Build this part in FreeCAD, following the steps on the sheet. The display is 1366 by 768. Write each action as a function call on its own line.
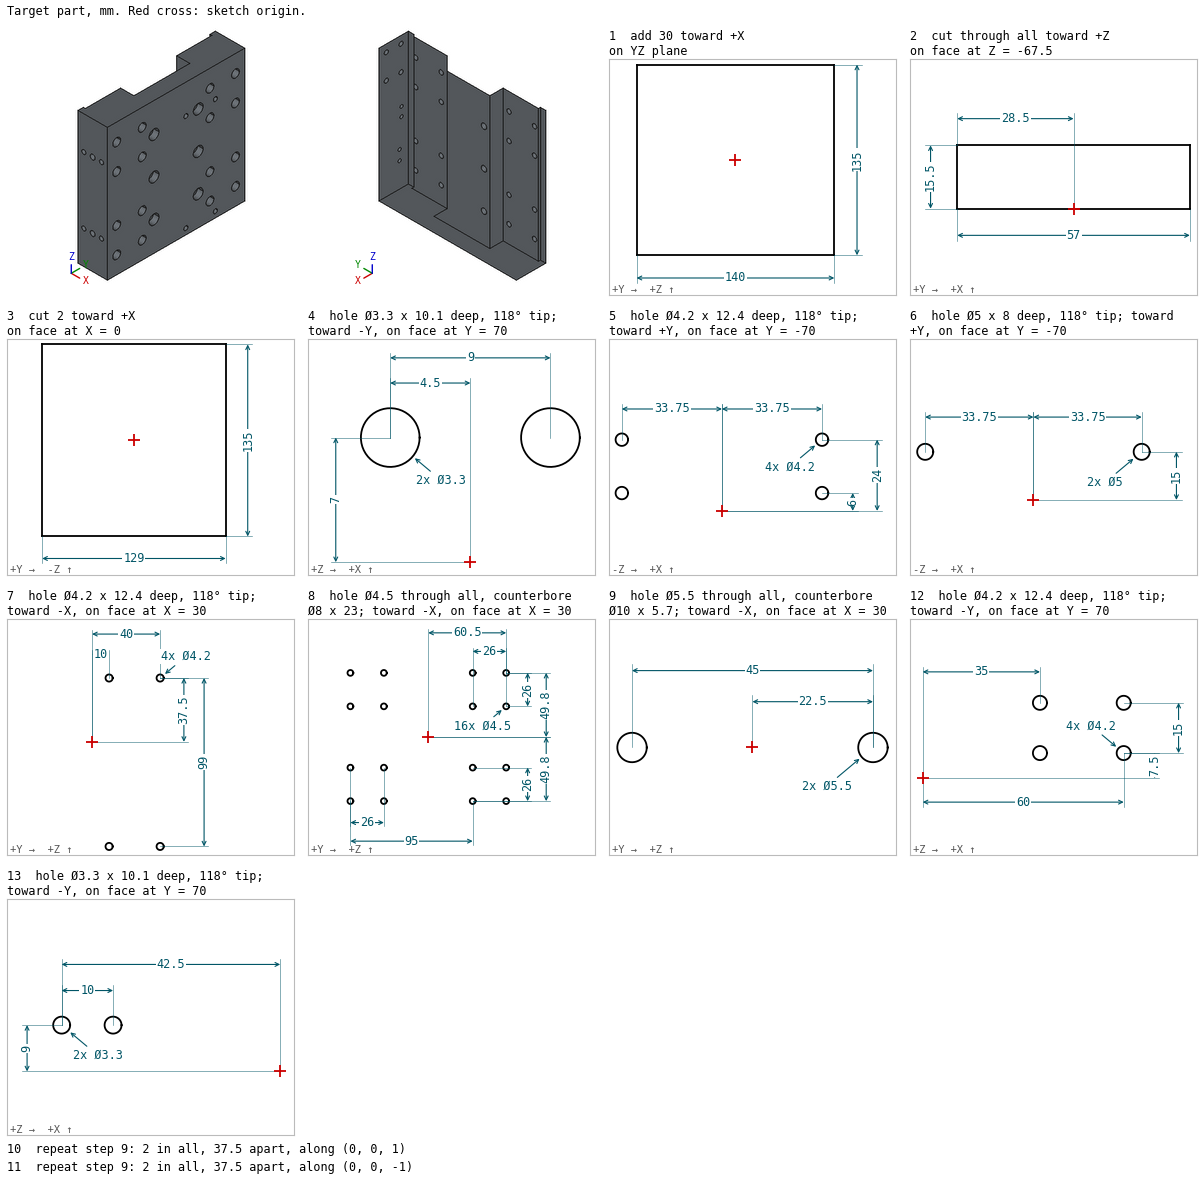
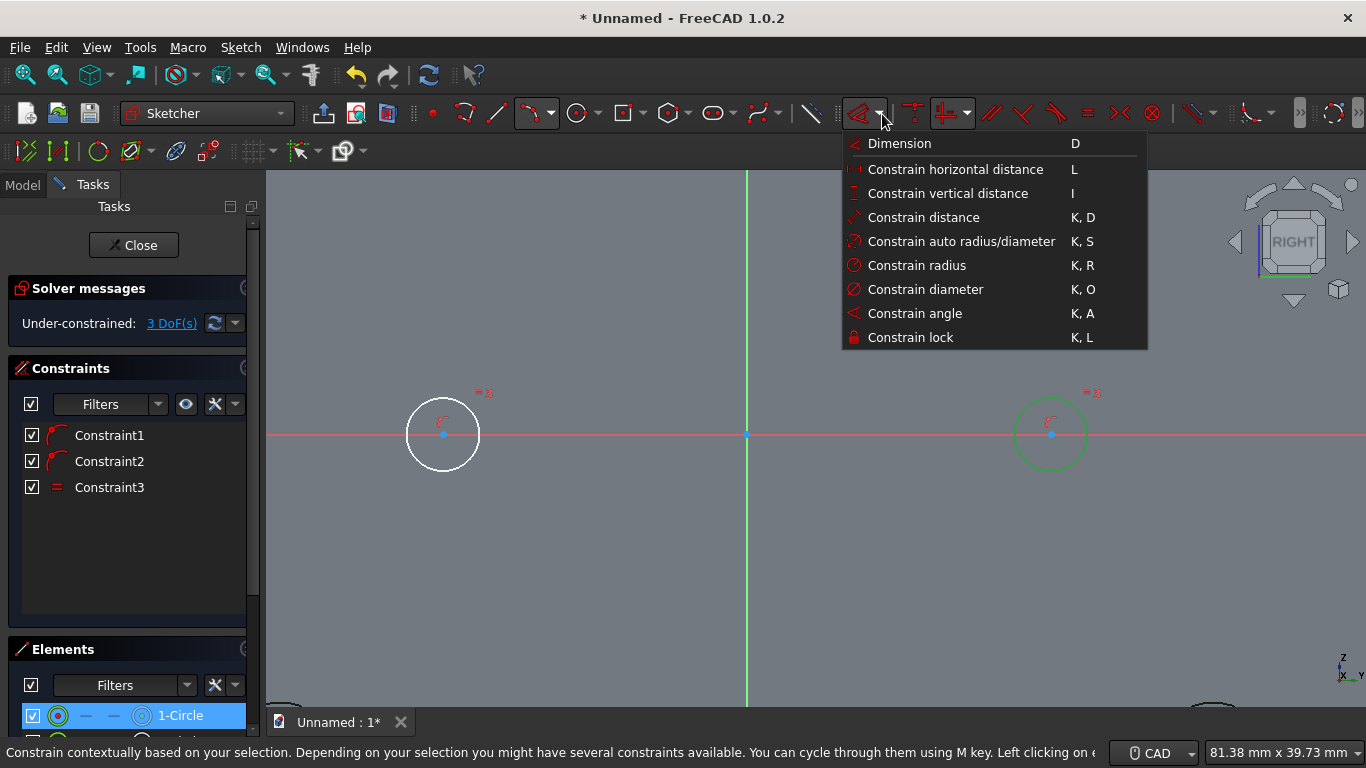
click(995, 289)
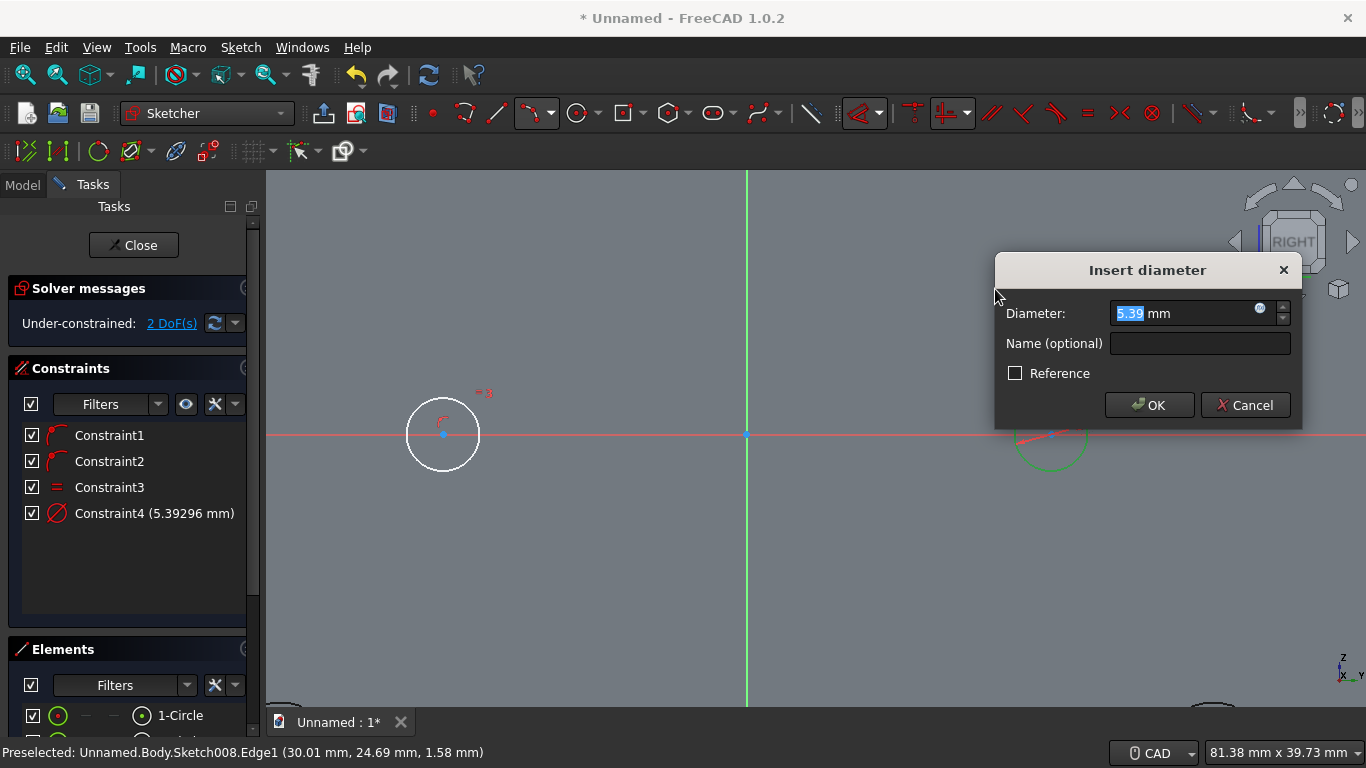
text(5.5)
key(Return)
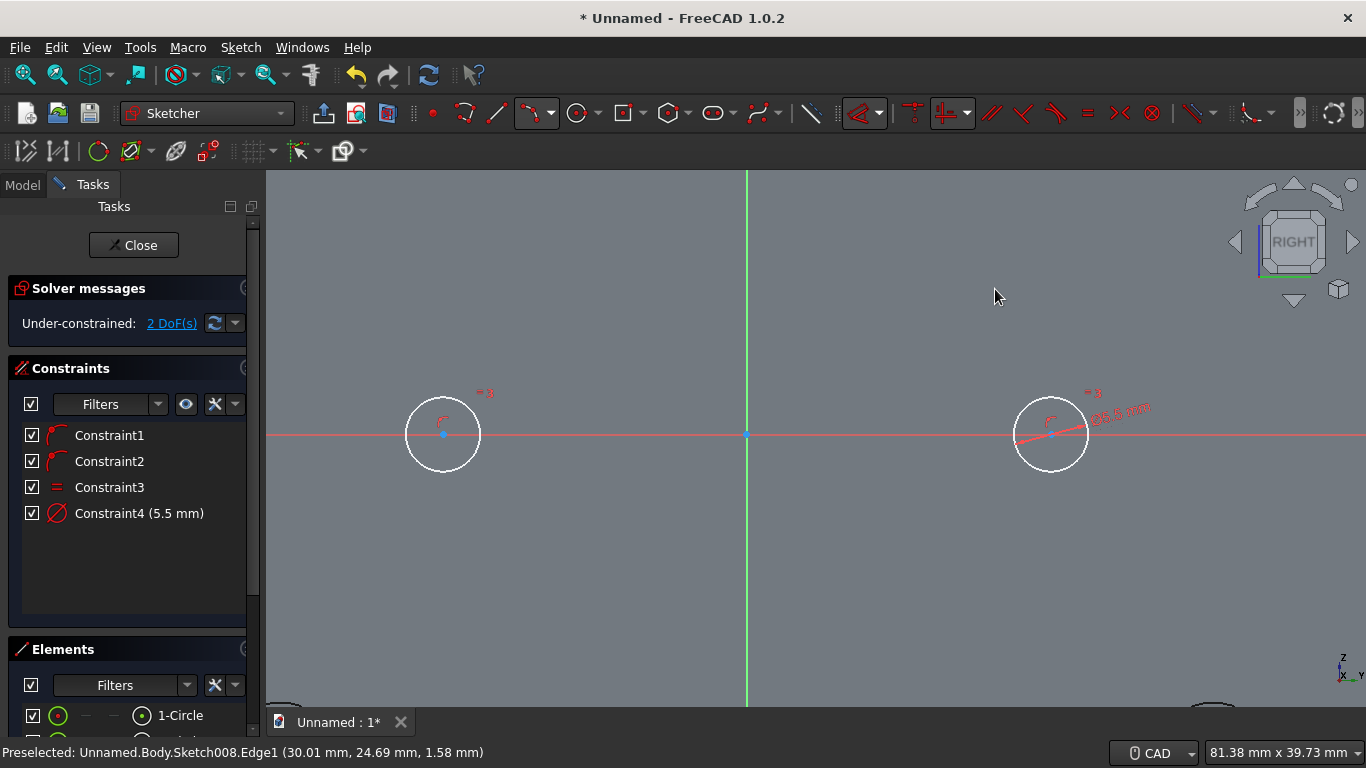
click(1051, 435)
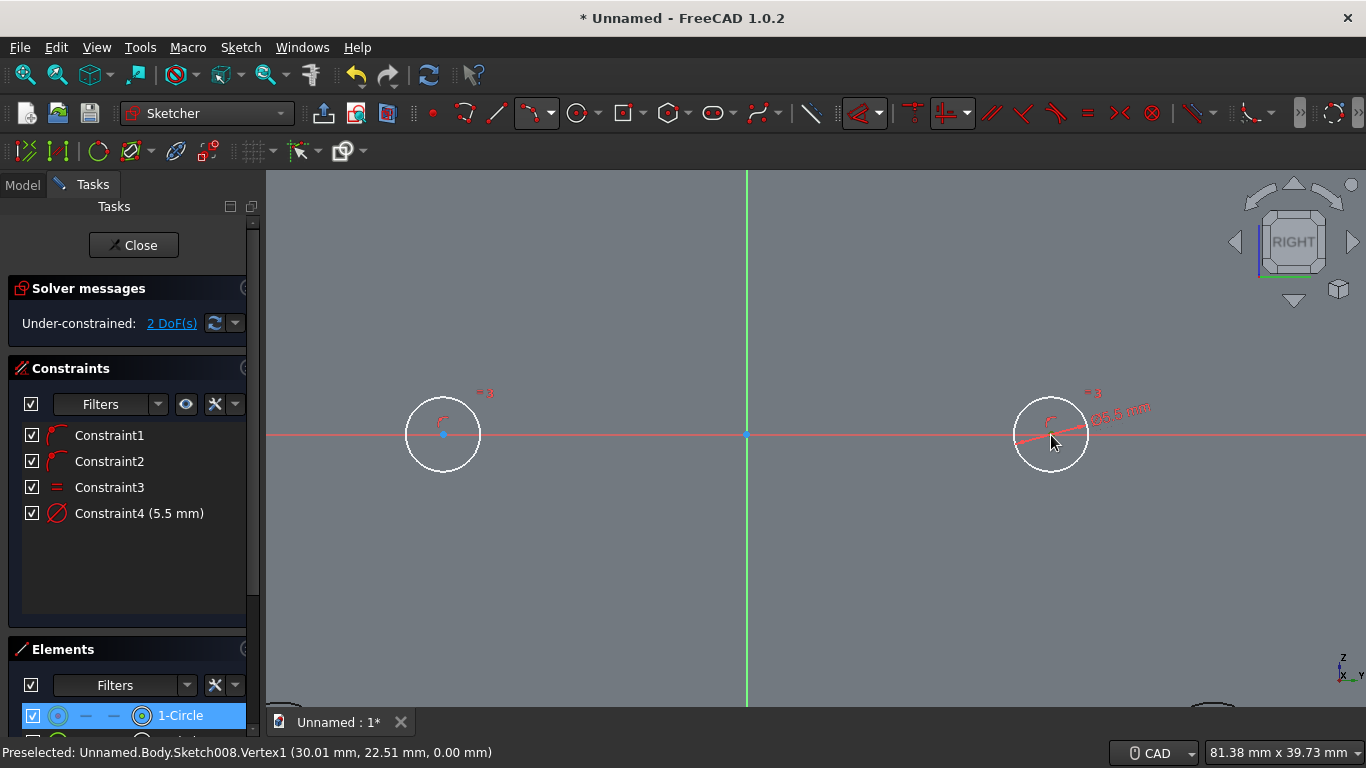
click(443, 435)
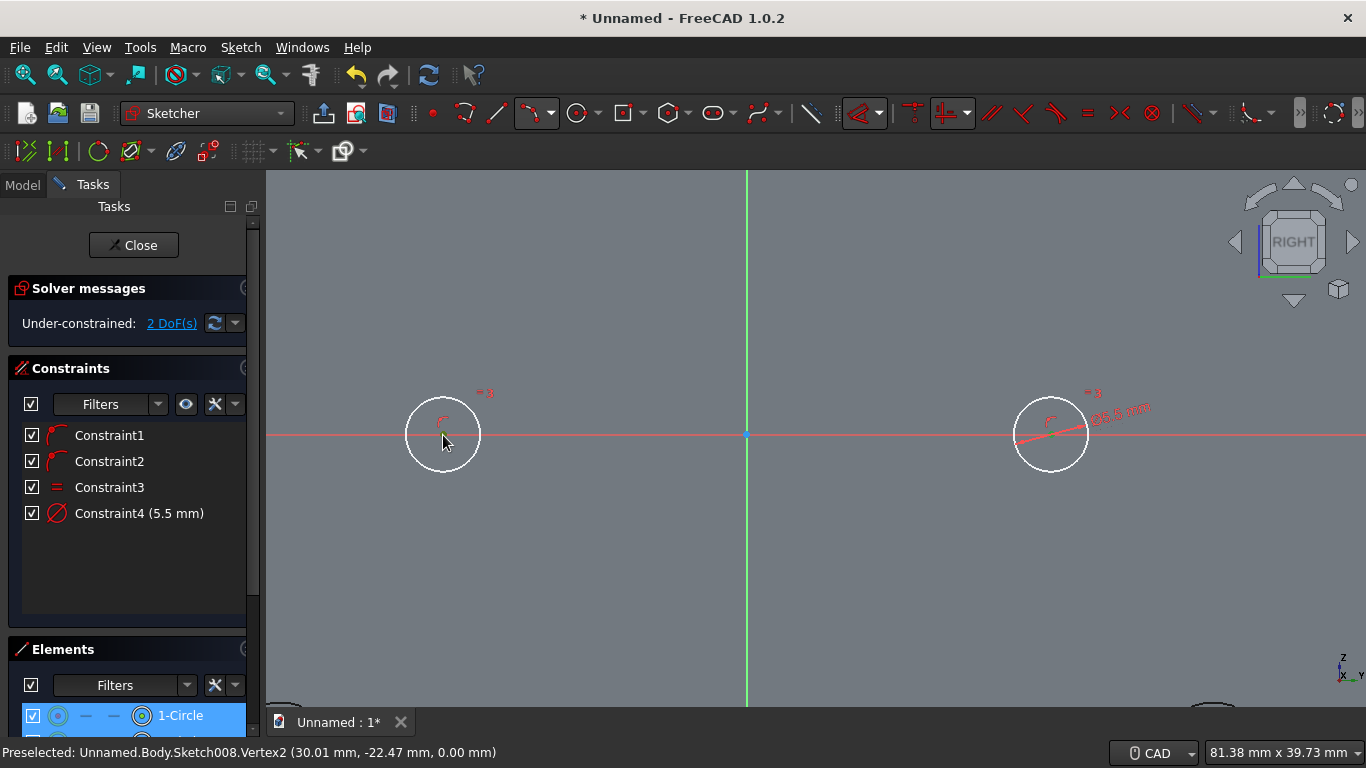
click(882, 114)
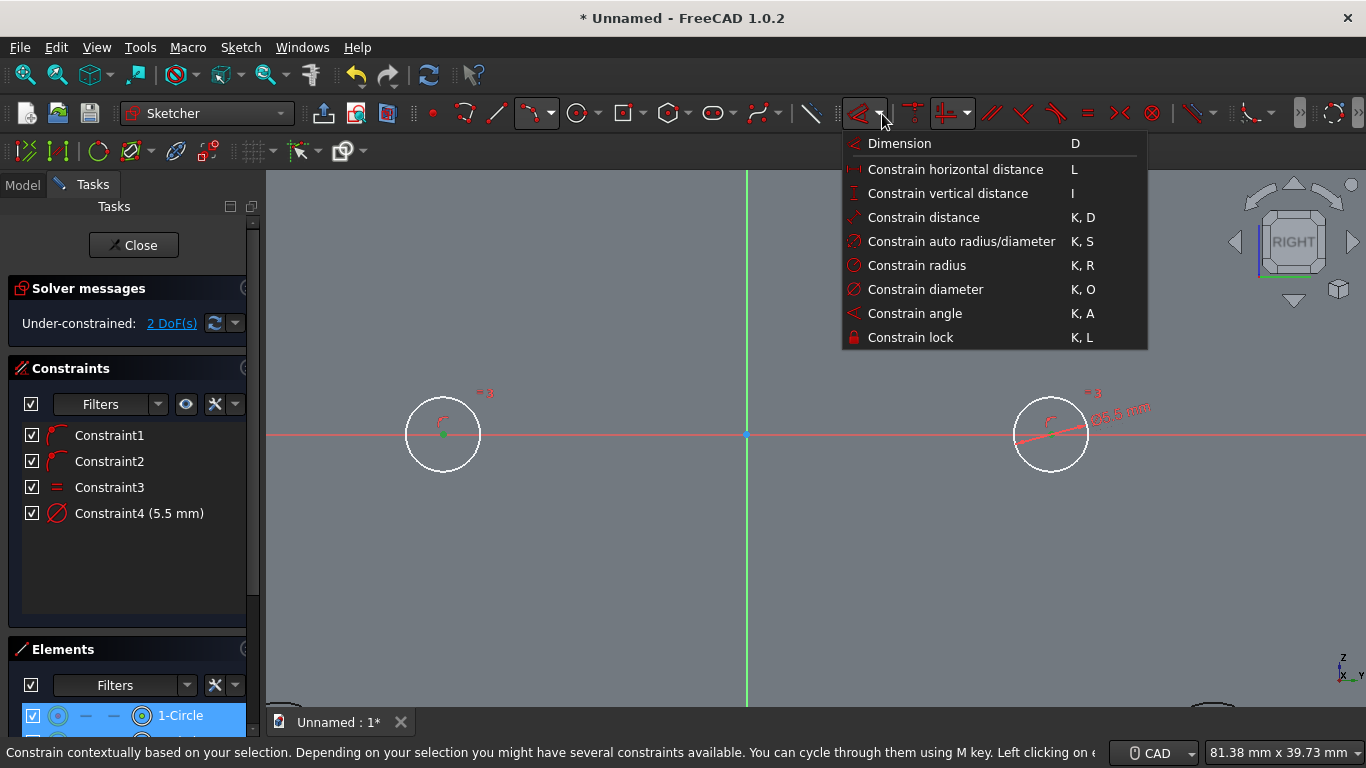
click(995, 169)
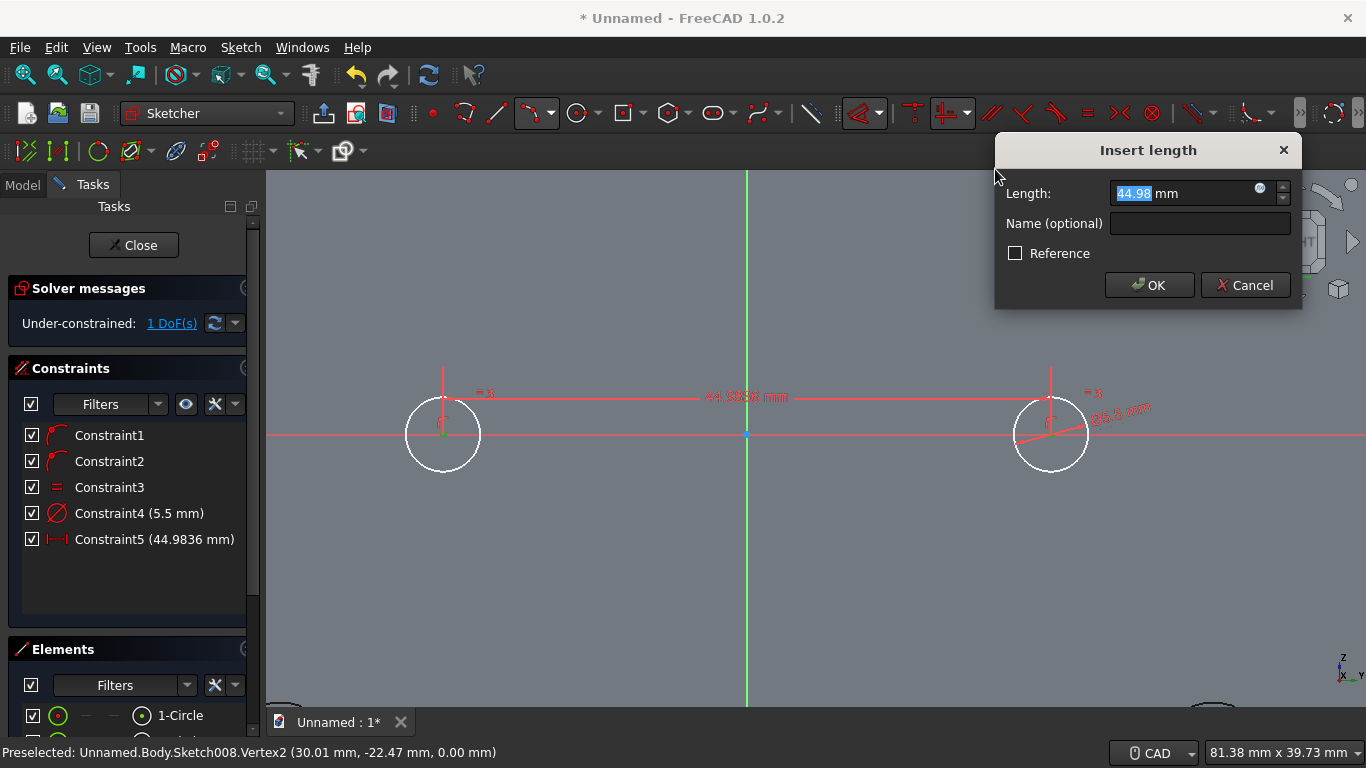
text(45)
key(Return)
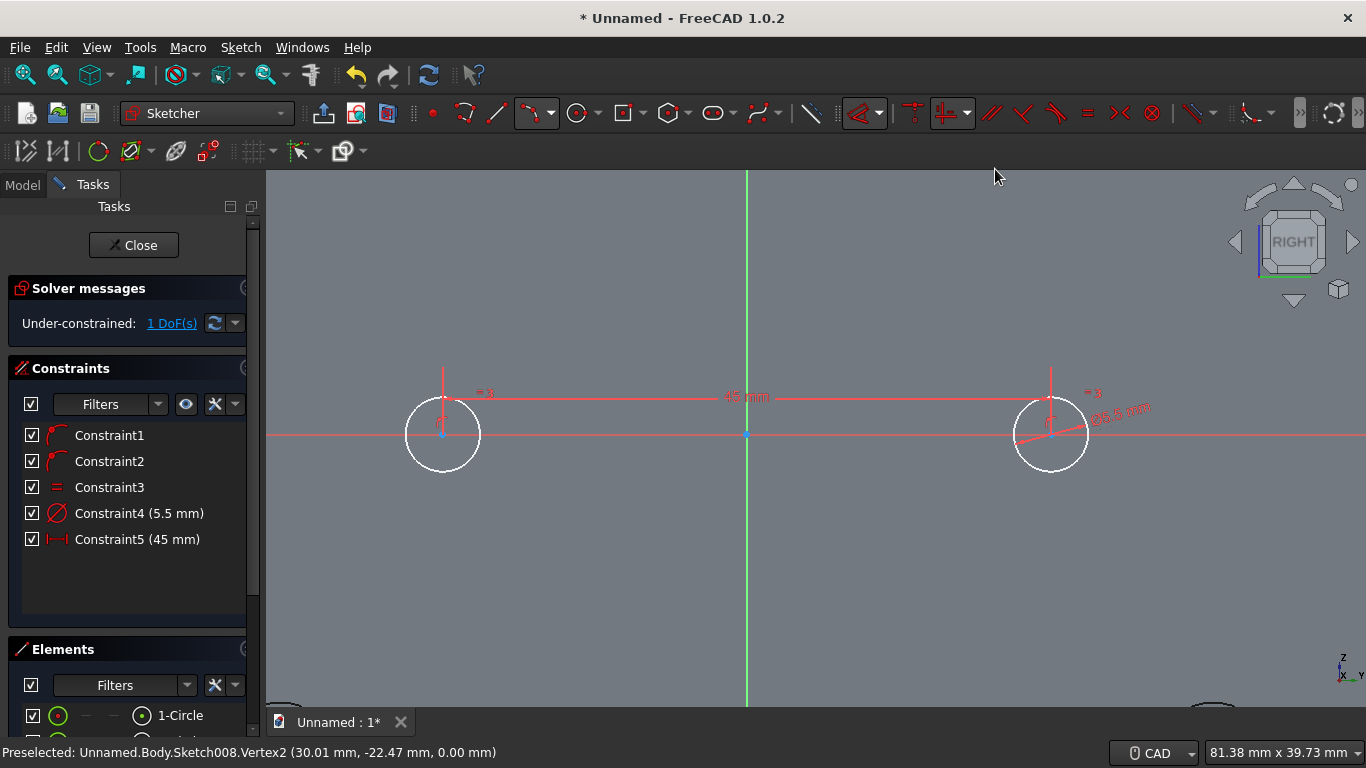
click(1051, 435)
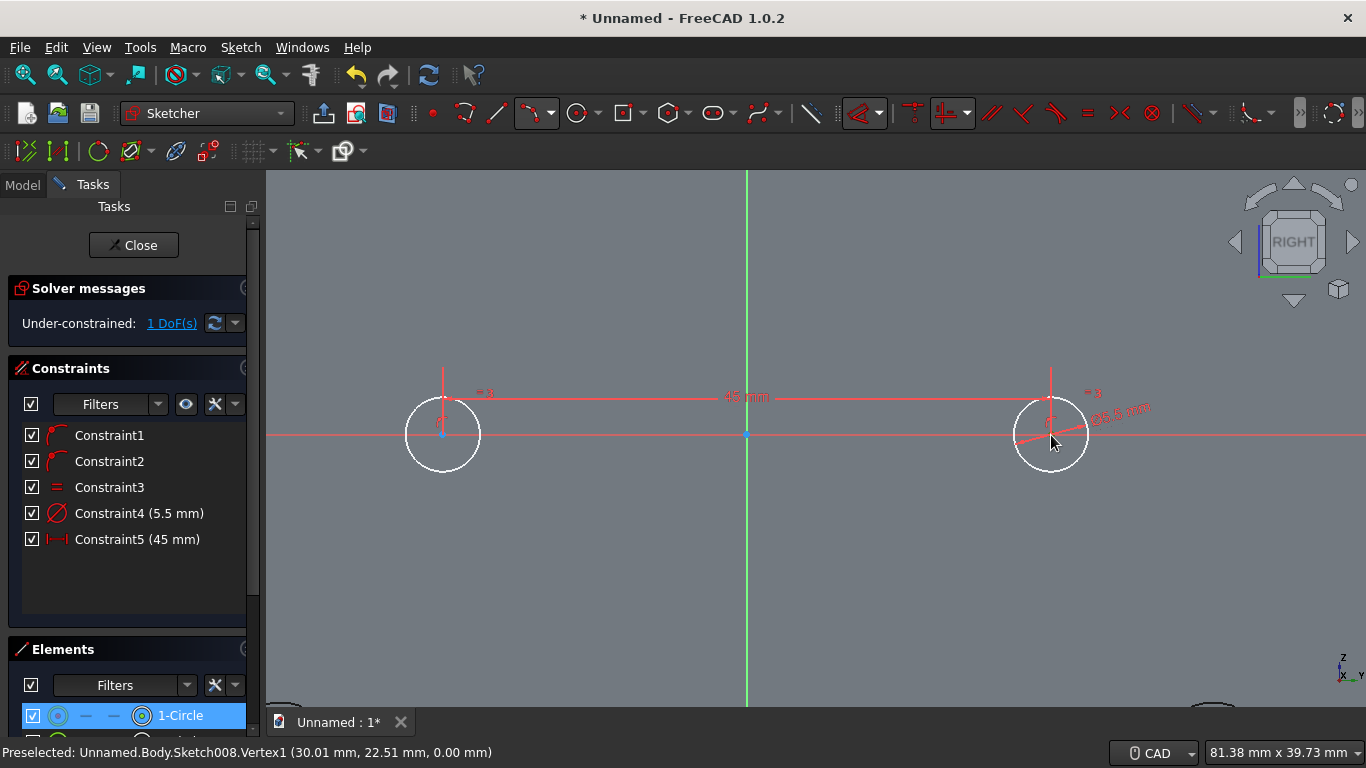
click(882, 114)